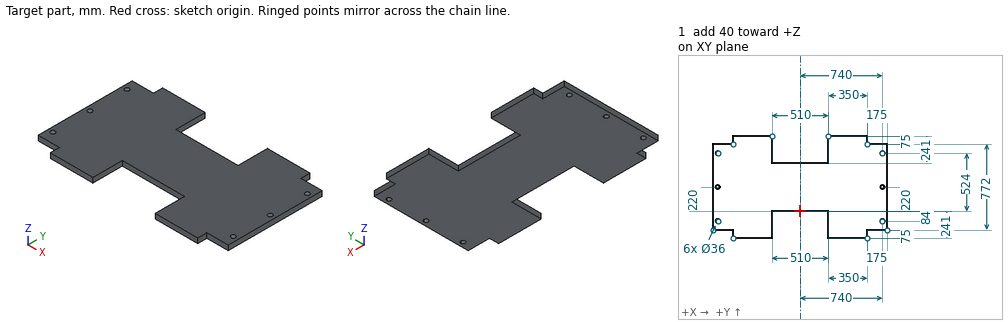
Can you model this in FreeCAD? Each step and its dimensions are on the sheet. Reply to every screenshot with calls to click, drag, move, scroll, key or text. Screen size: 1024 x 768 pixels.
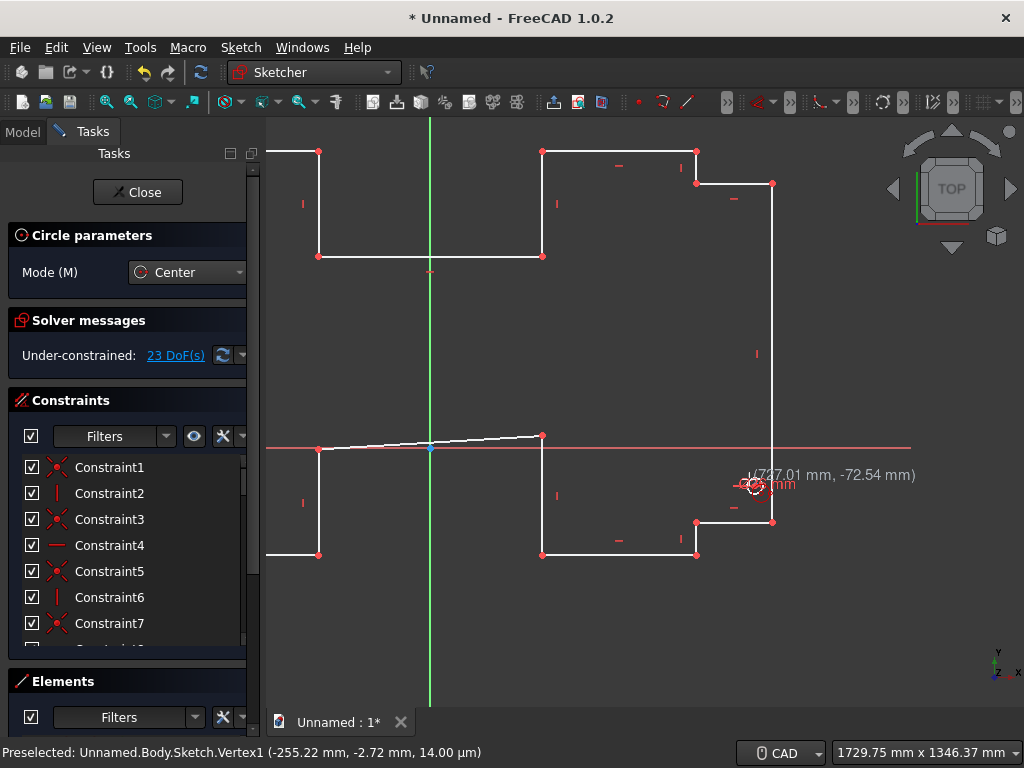
scroll(755, 352, up, 6)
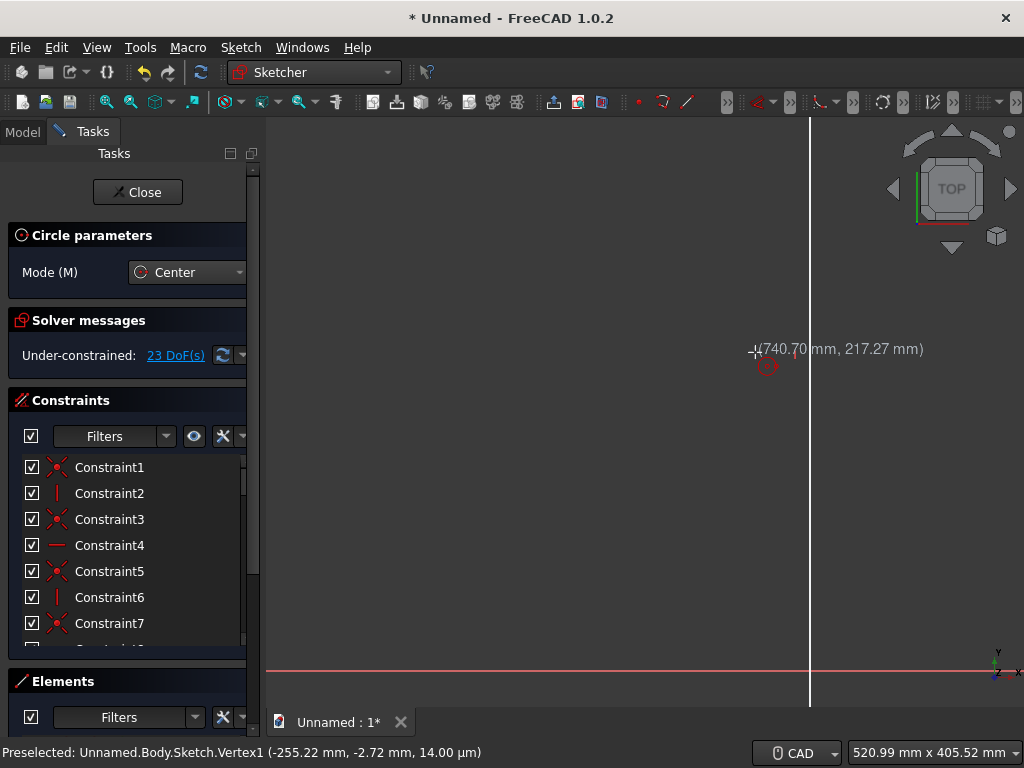
scroll(755, 424, down, 9)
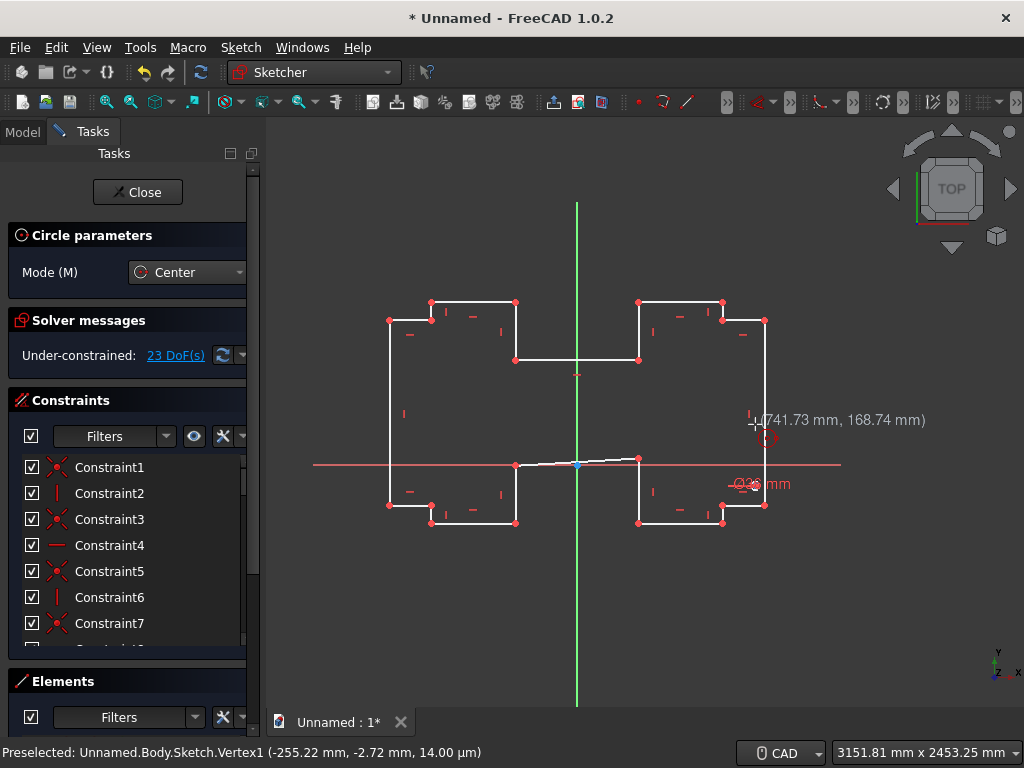
scroll(755, 412, up, 3)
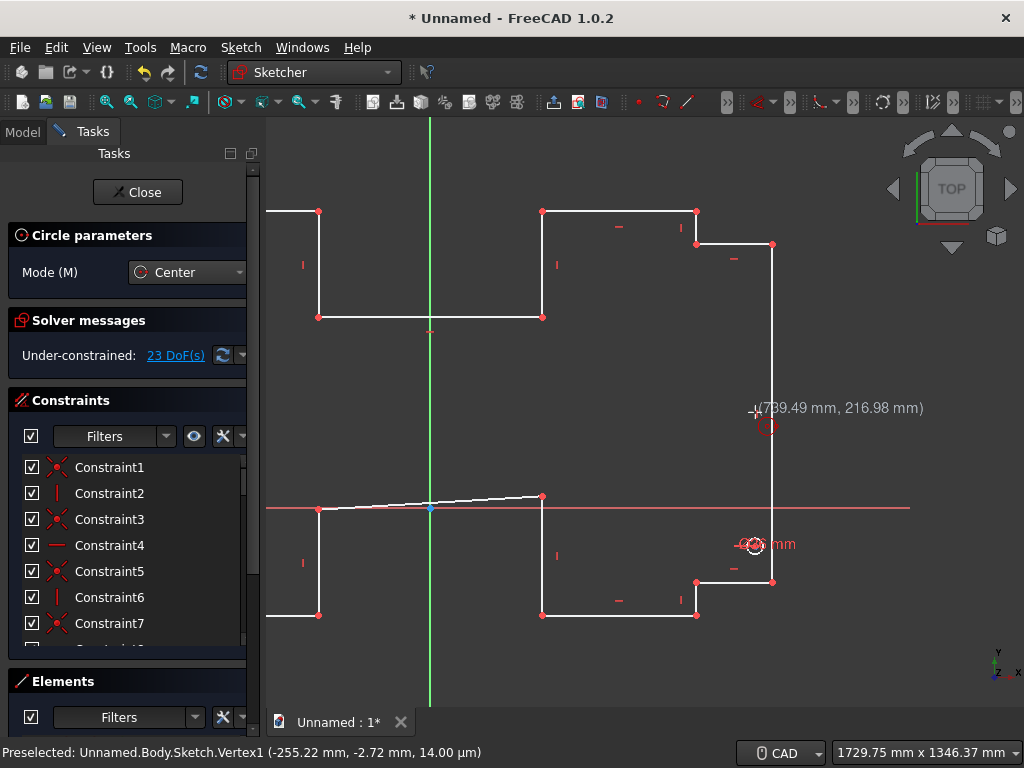
click(755, 412)
move(749, 407)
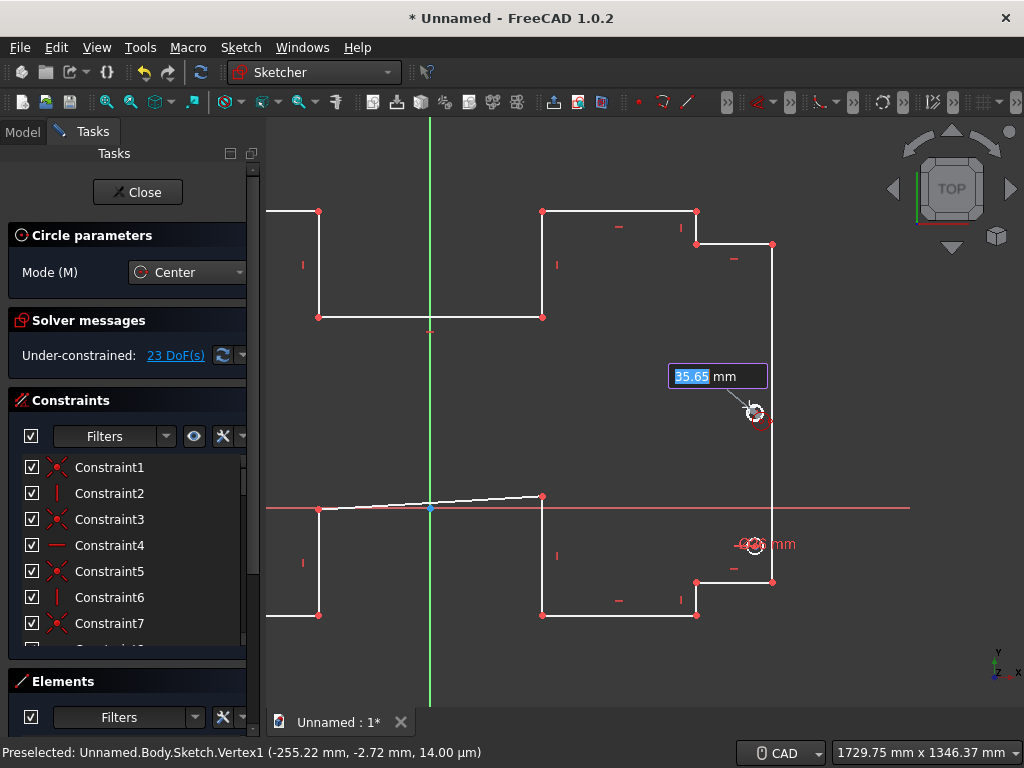
text(36)
key(Return)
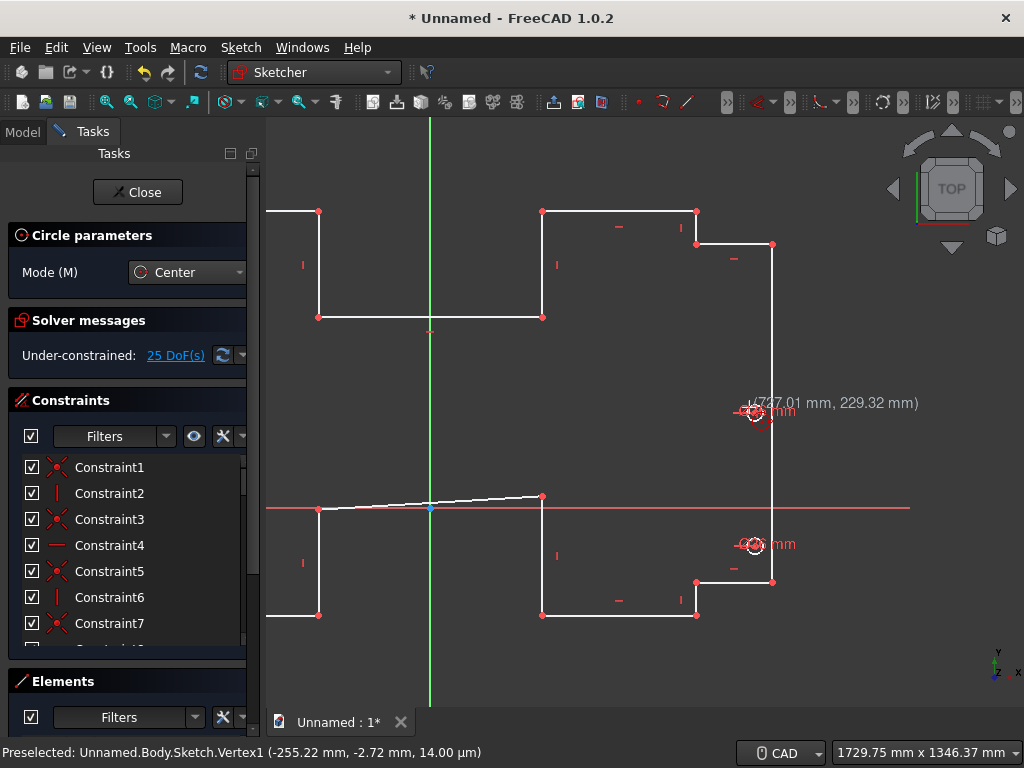
scroll(754, 412, down, 3)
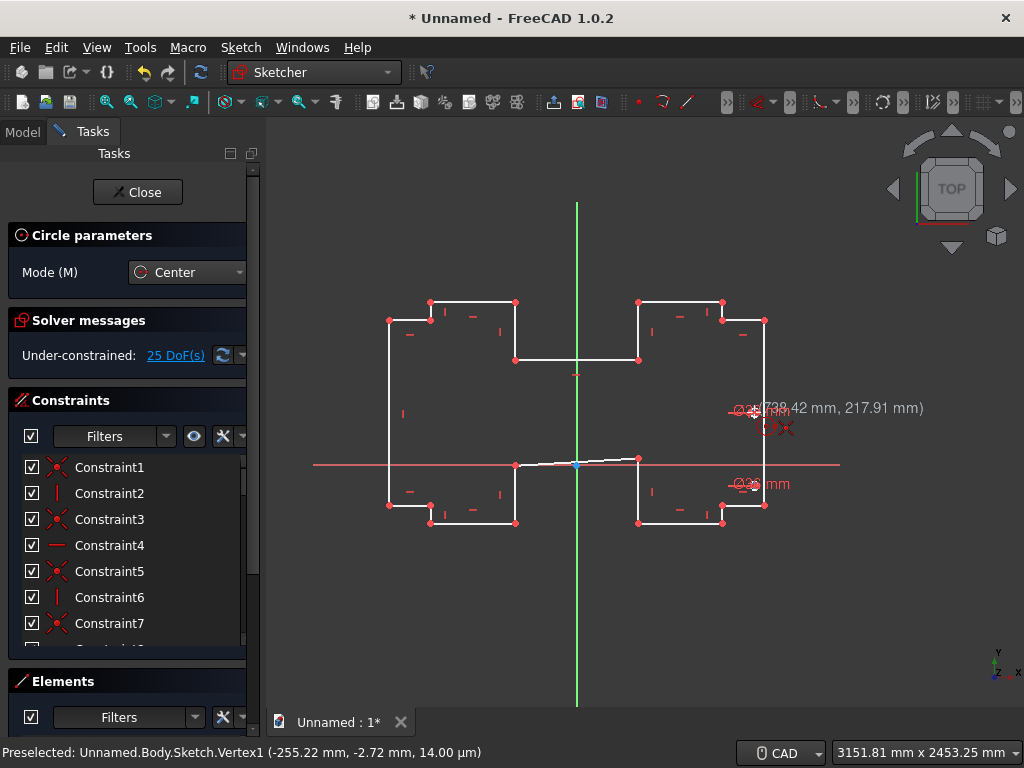
scroll(399, 485, up, 9)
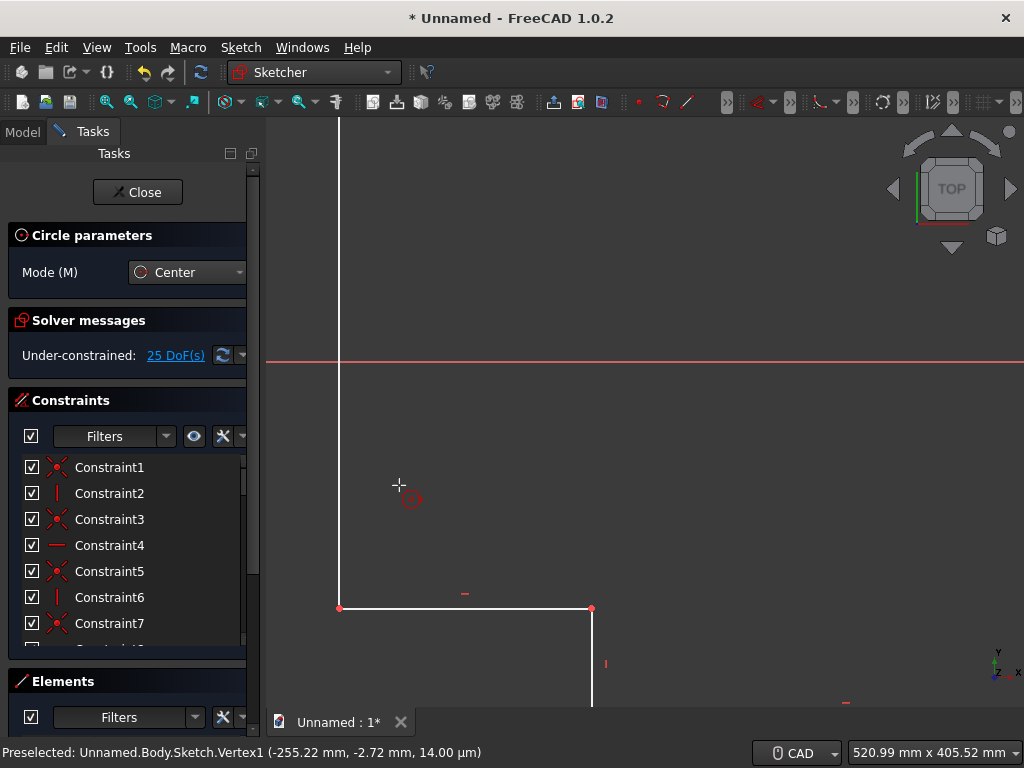
scroll(399, 485, down, 9)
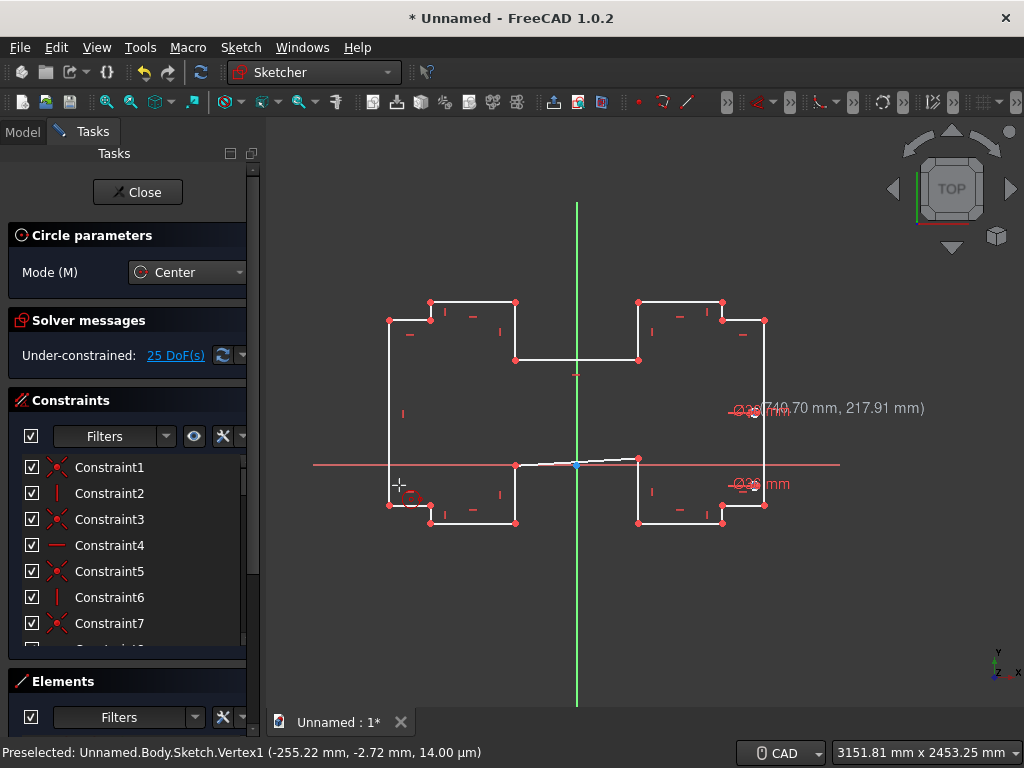
scroll(399, 485, up, 3)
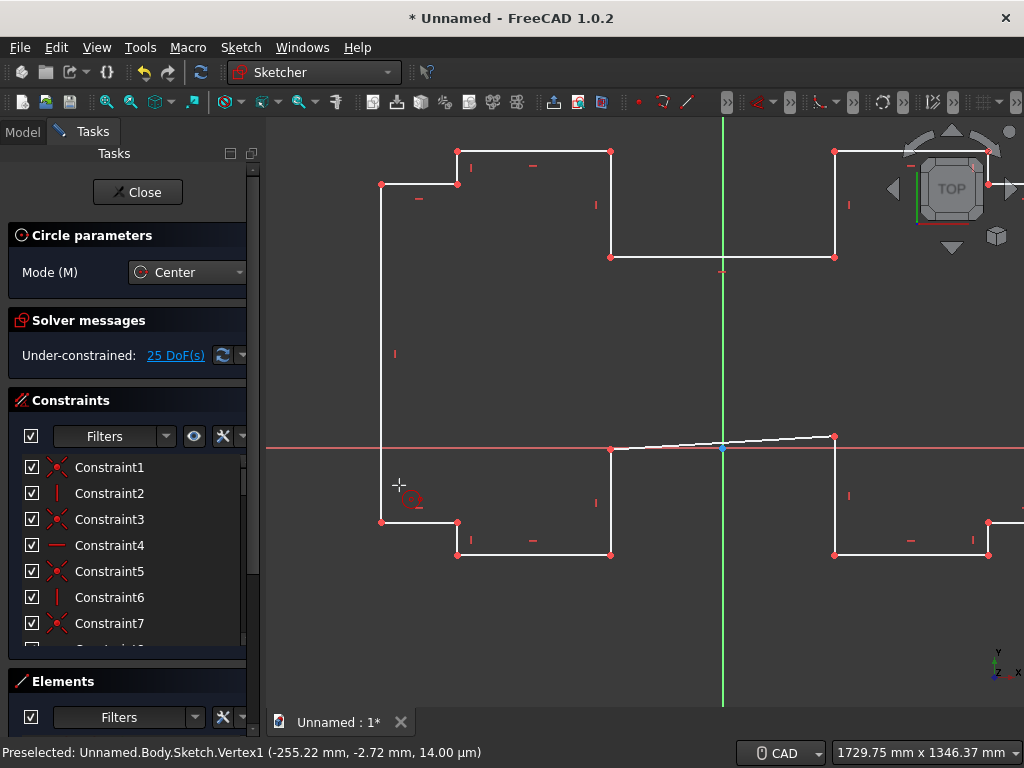
click(398, 485)
move(404, 480)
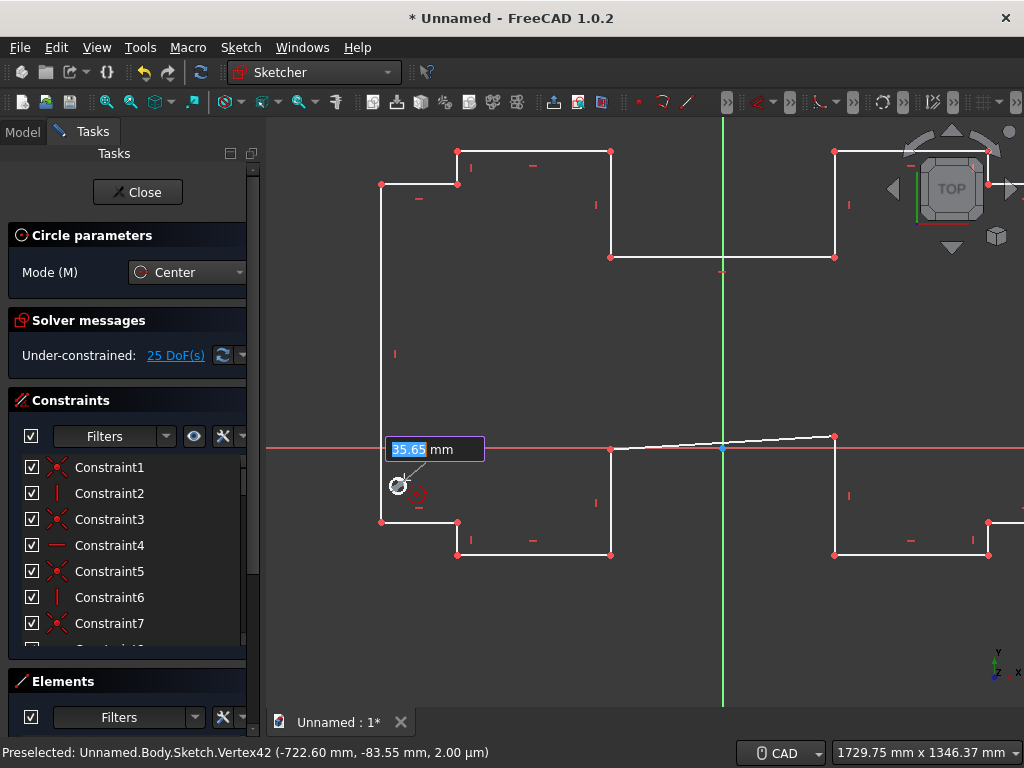
text(36)
key(Return)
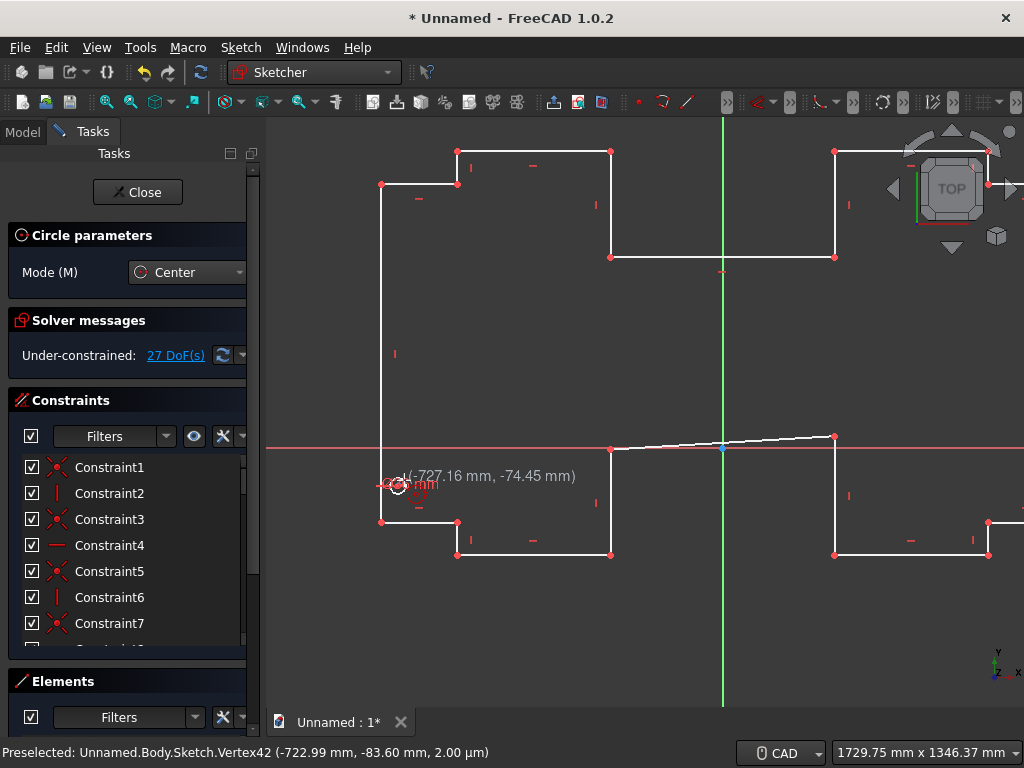
scroll(398, 352, up, 6)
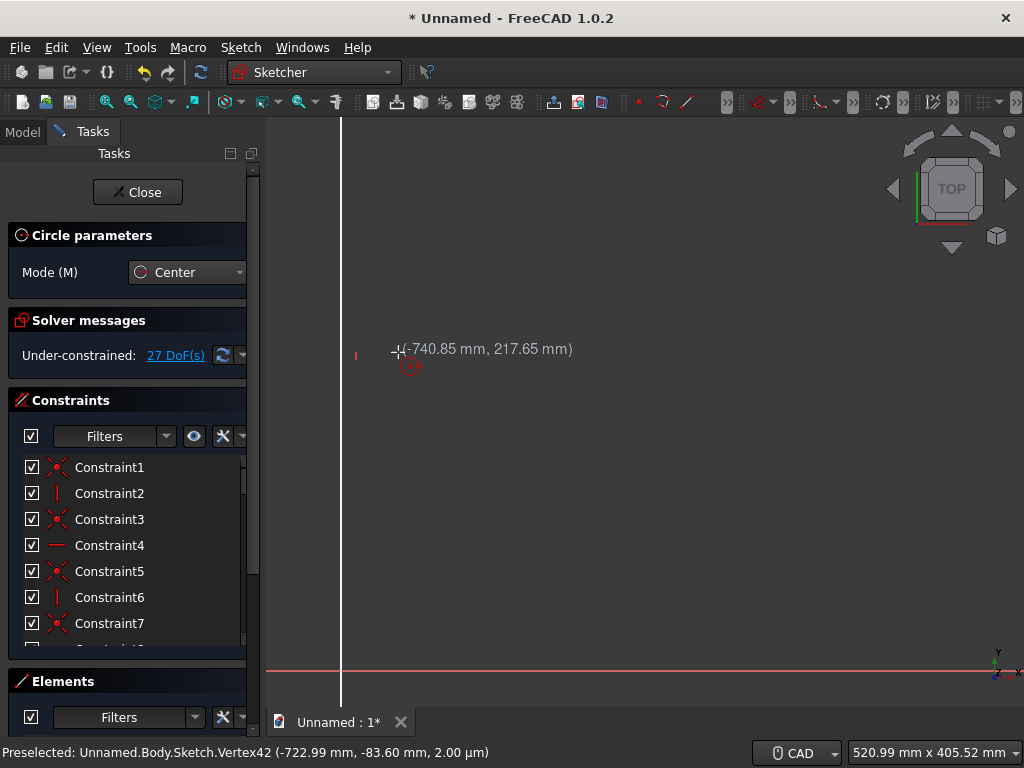
scroll(398, 424, down, 9)